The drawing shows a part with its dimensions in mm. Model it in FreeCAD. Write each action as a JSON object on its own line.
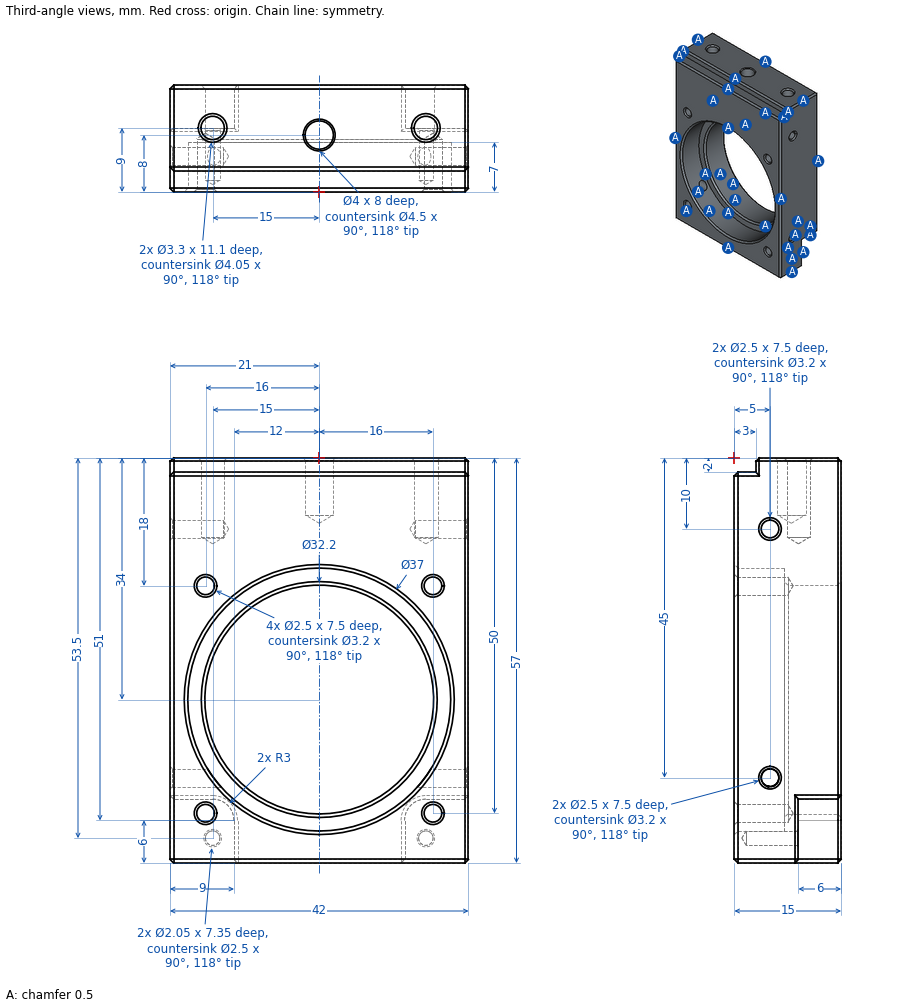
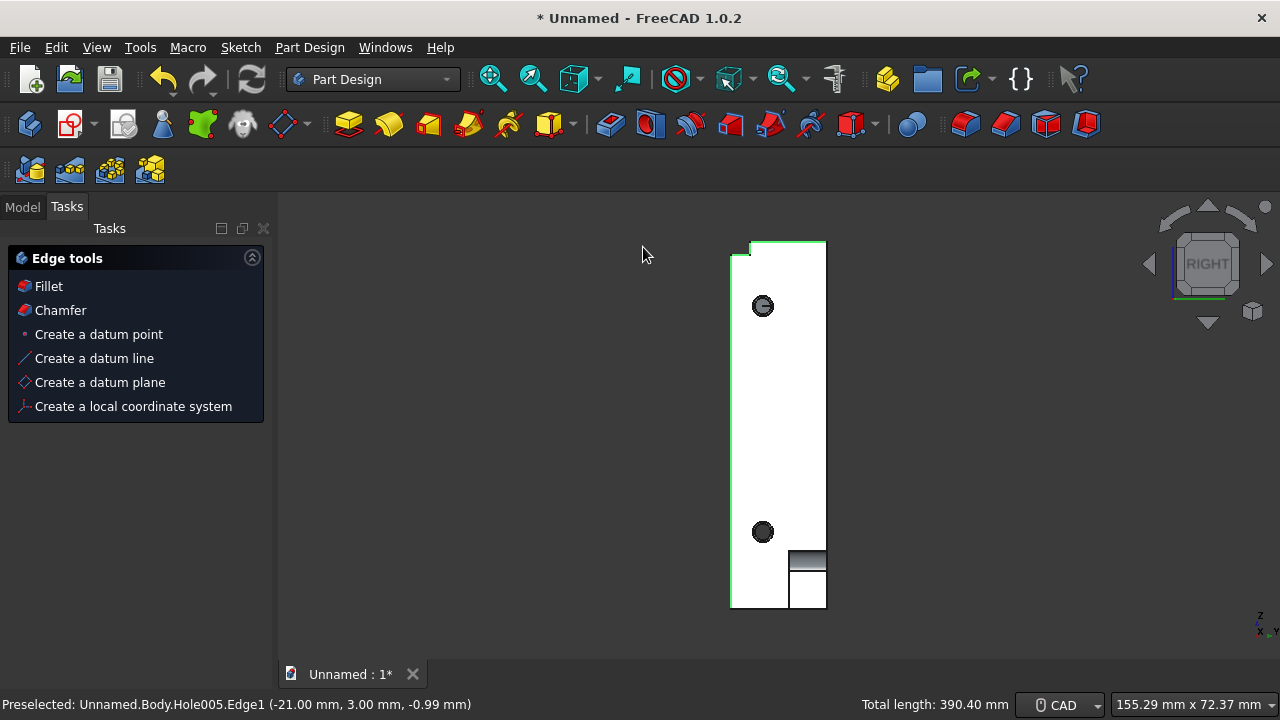
{"action": "left_click", "coordinate": [789, 579], "text": "ctrl"}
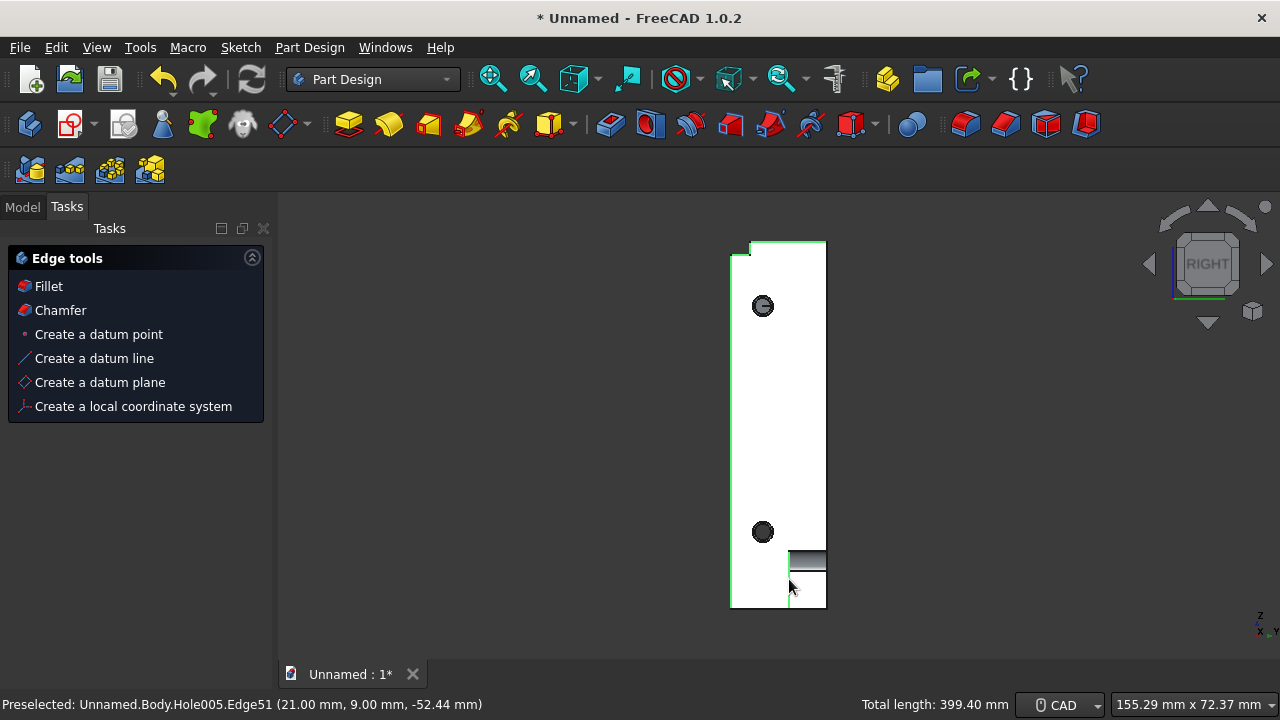
{"action": "left_click", "coordinate": [808, 550], "text": "ctrl"}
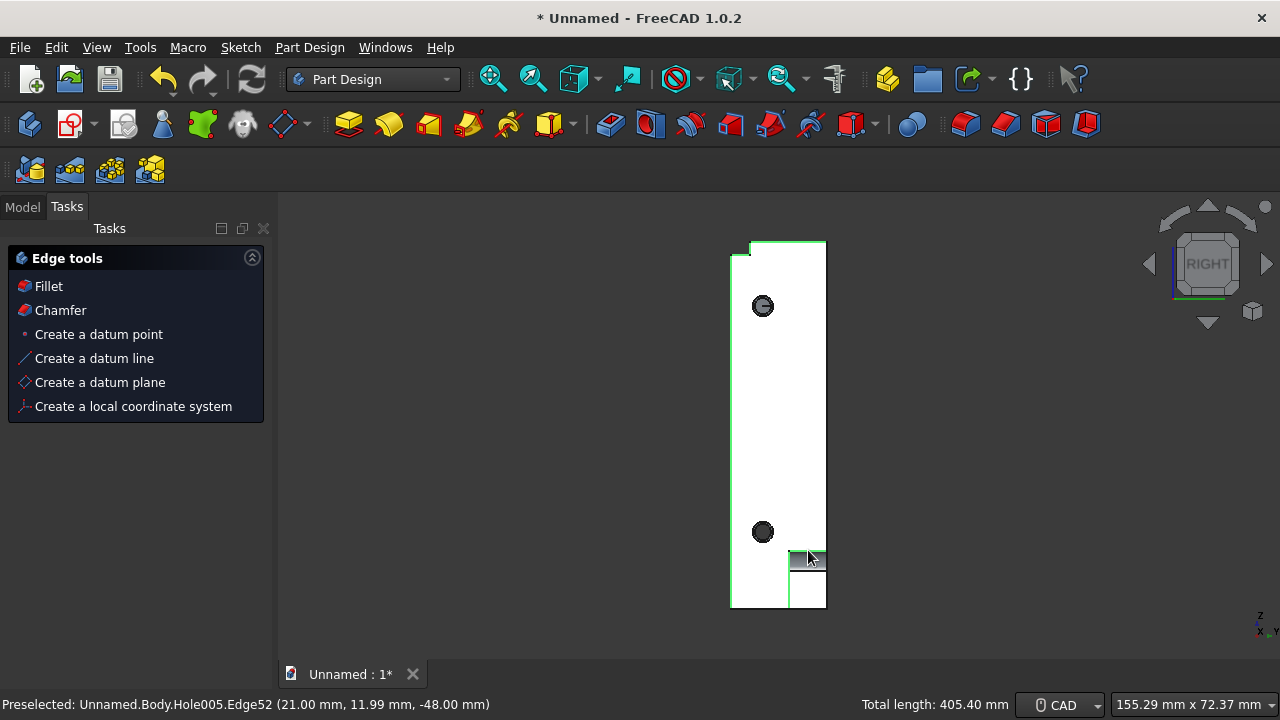
{"action": "key", "text": "5"}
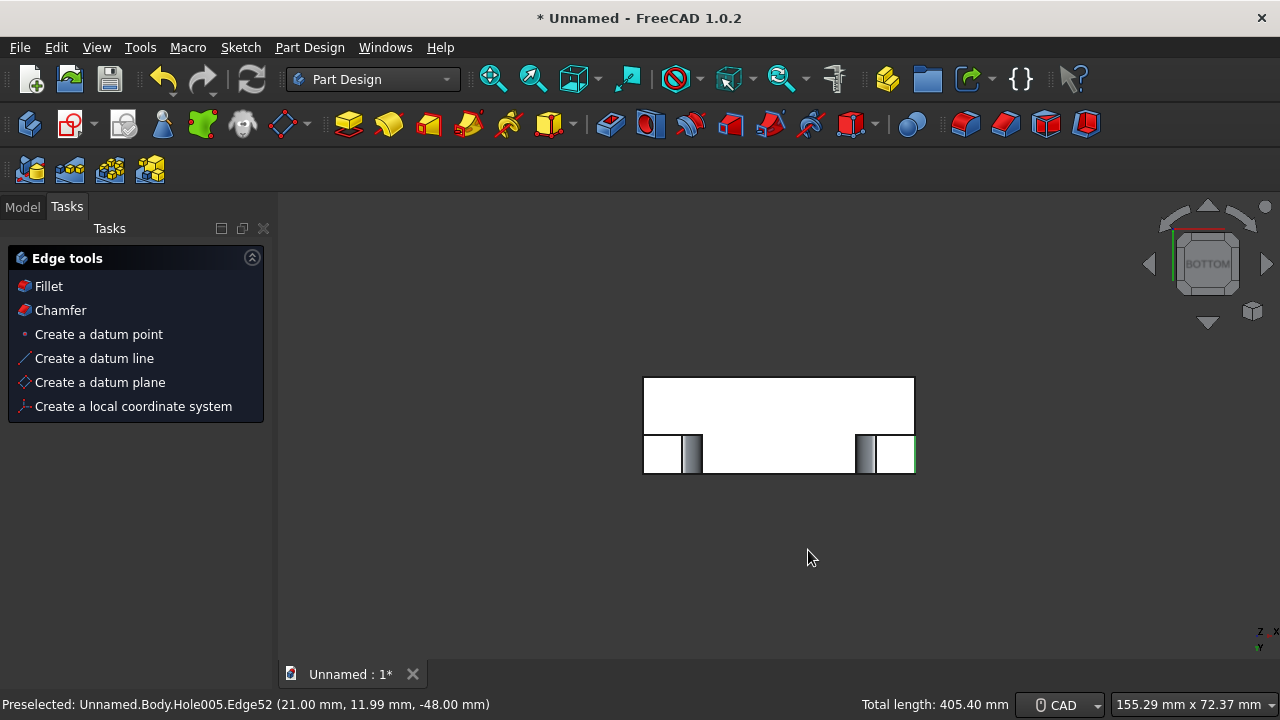
{"action": "key", "text": "v f"}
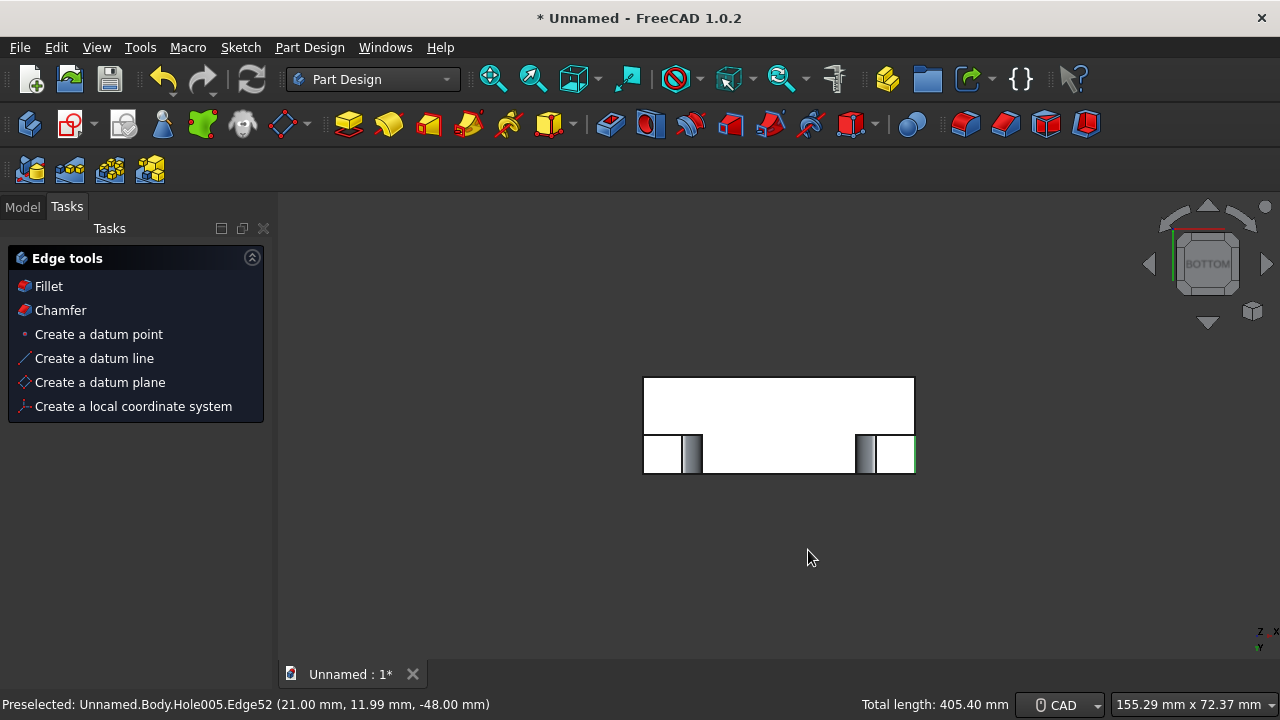
{"action": "left_click", "coordinate": [779, 424], "text": "ctrl"}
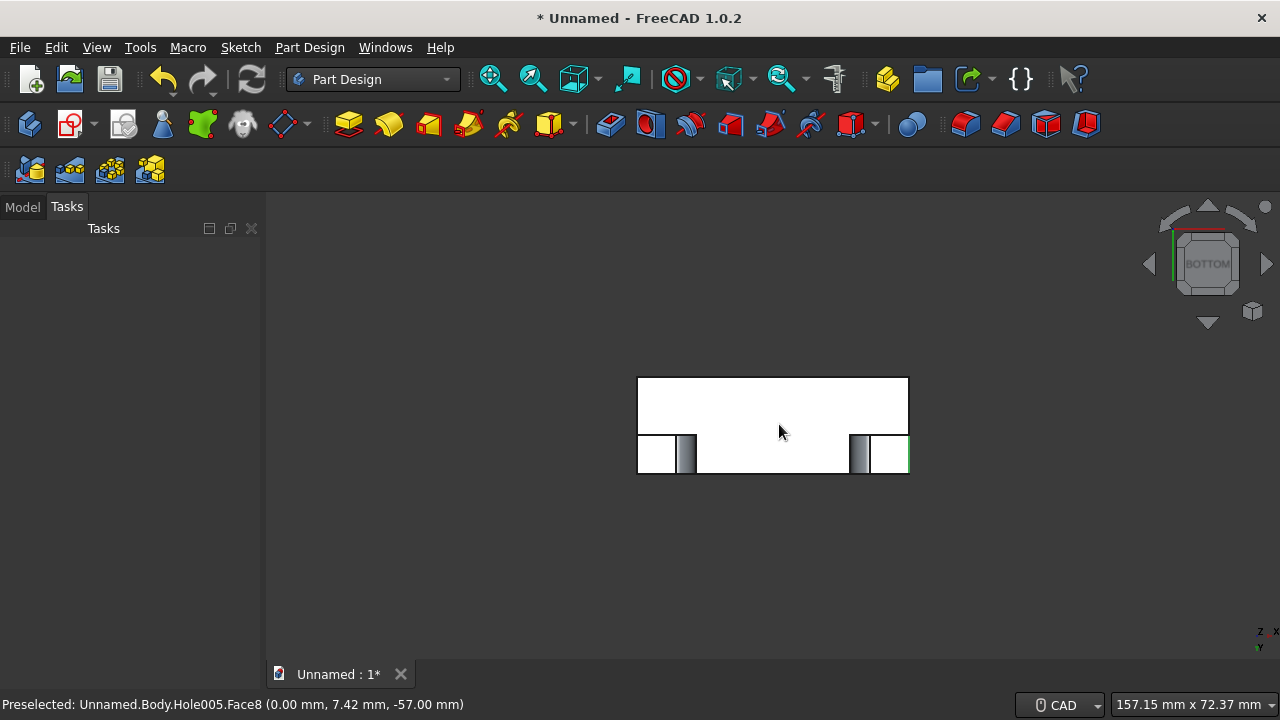
{"action": "left_click", "coordinate": [637, 454], "text": "ctrl"}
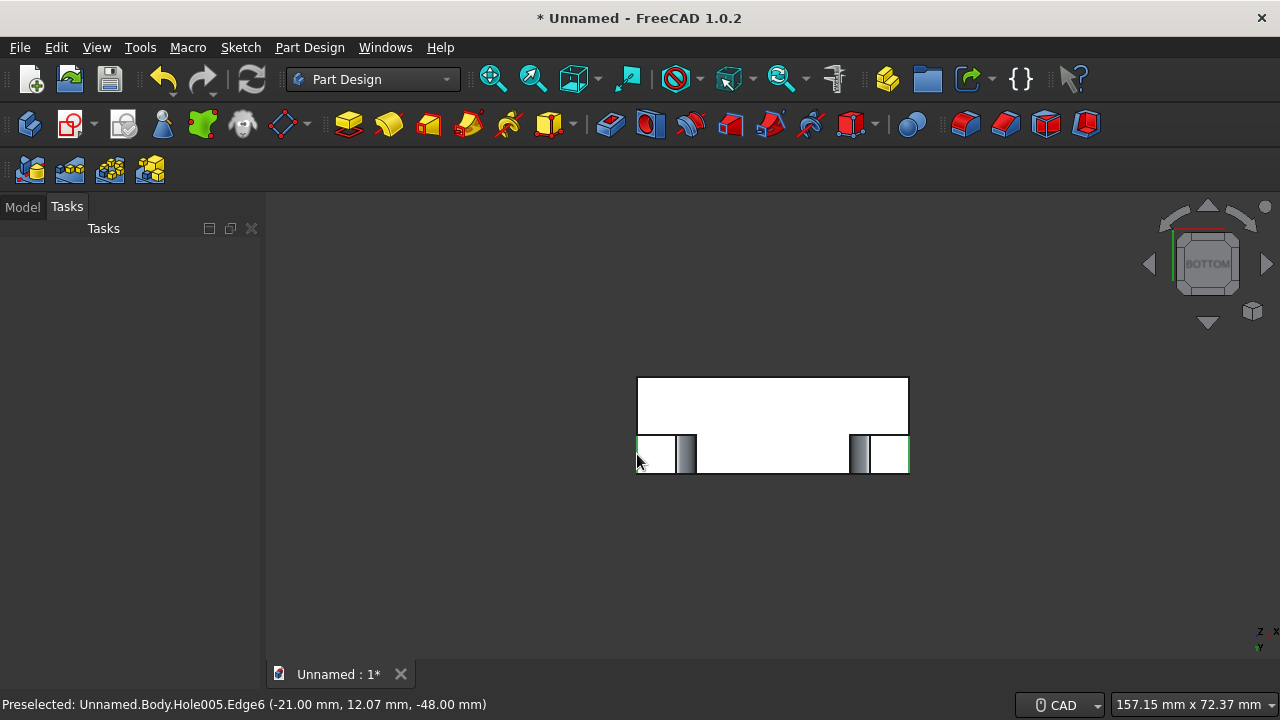
{"action": "key", "text": "4"}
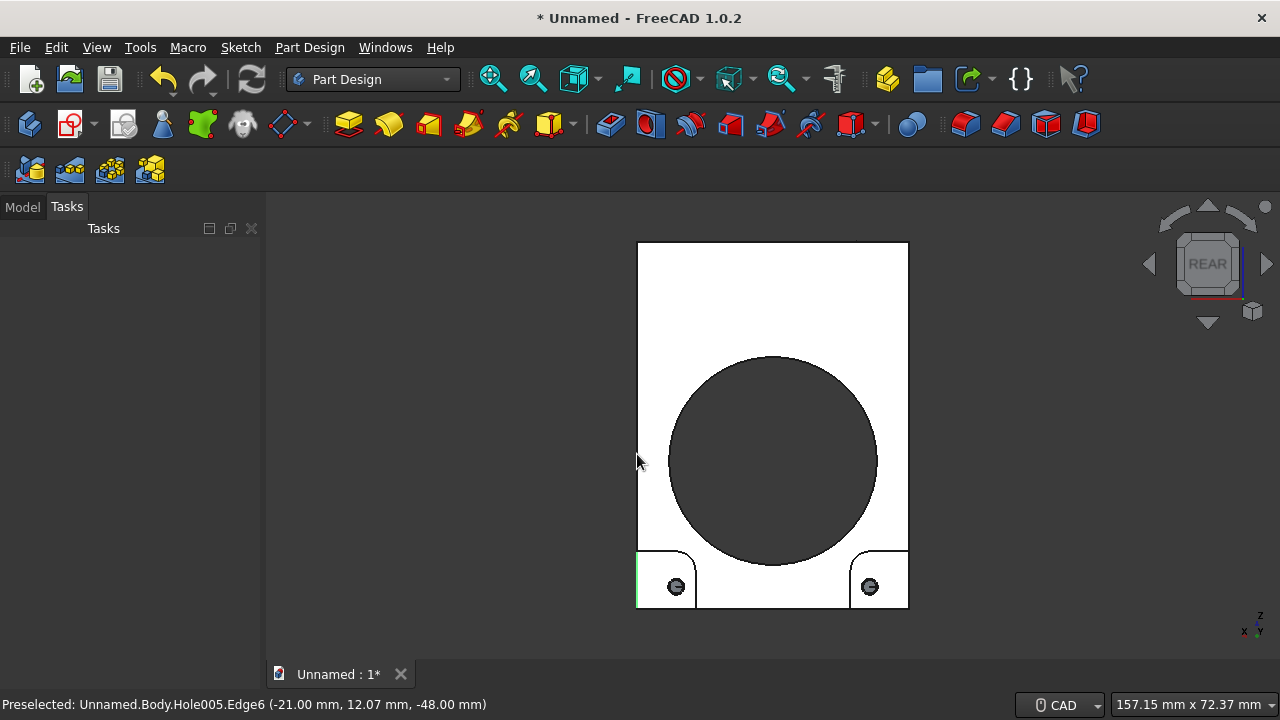
{"action": "left_click", "coordinate": [696, 319], "text": "ctrl"}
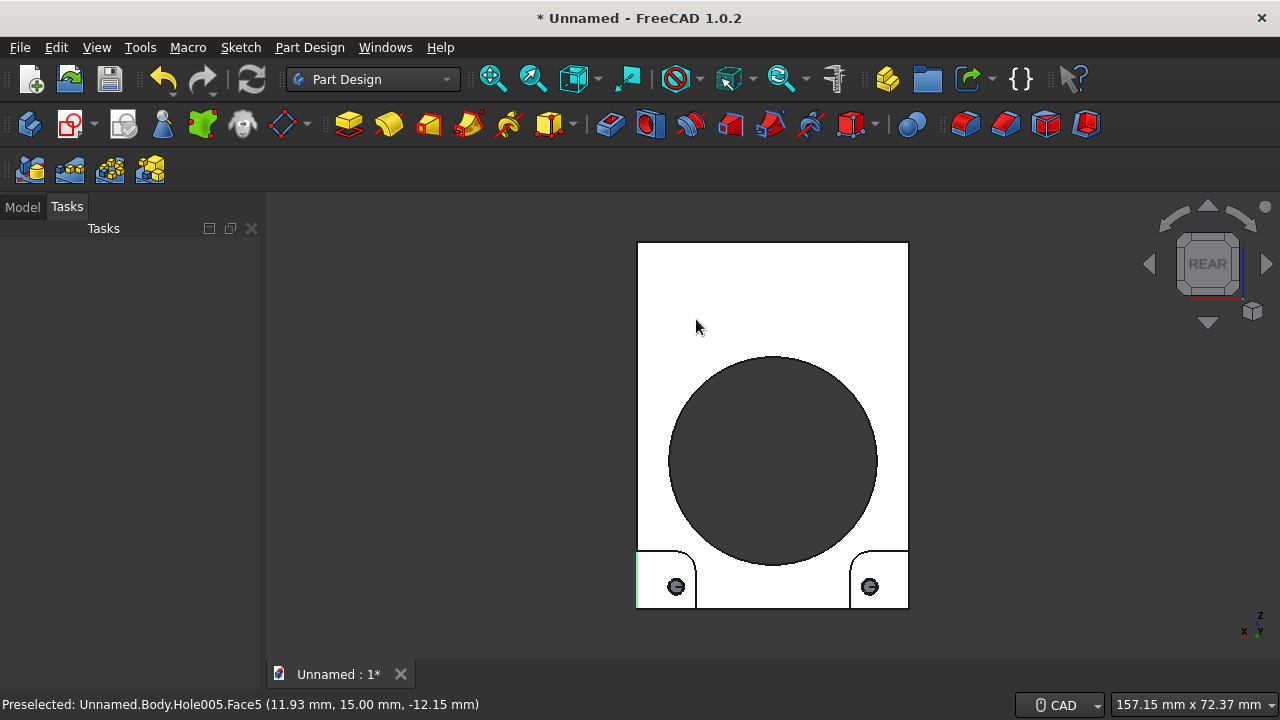
{"action": "left_click", "coordinate": [909, 579], "text": "ctrl"}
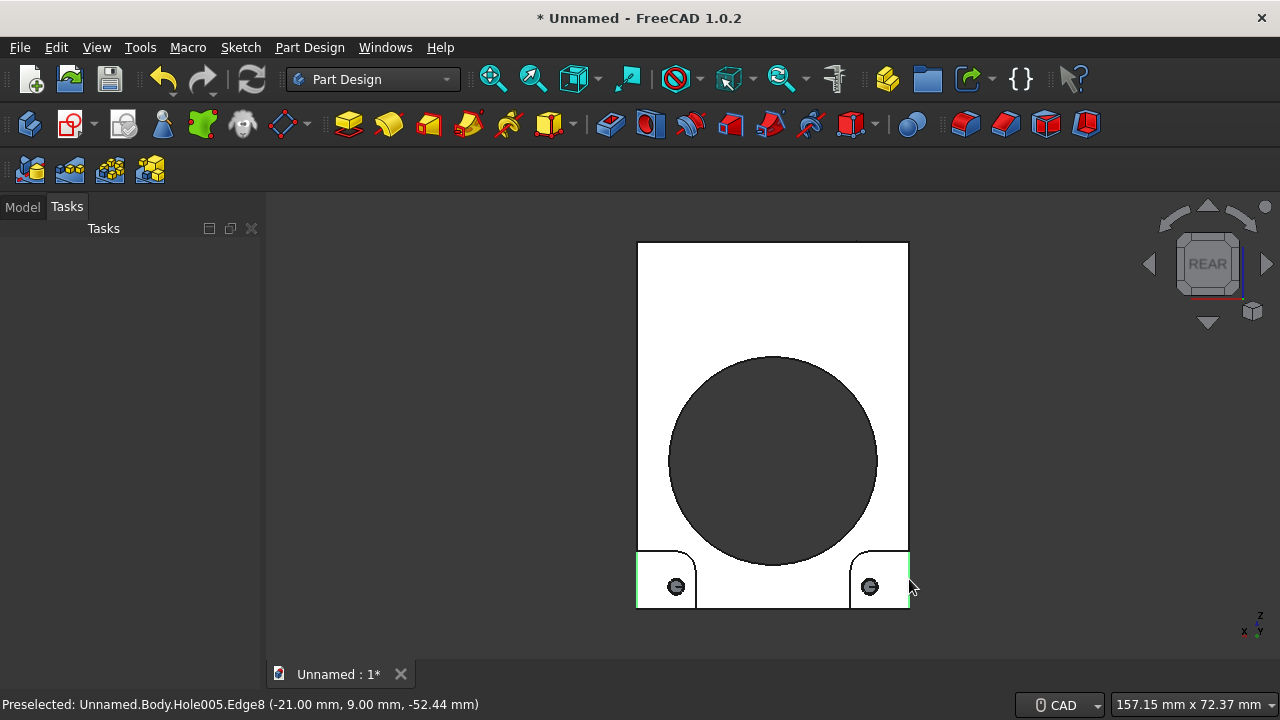
{"action": "key", "text": "6"}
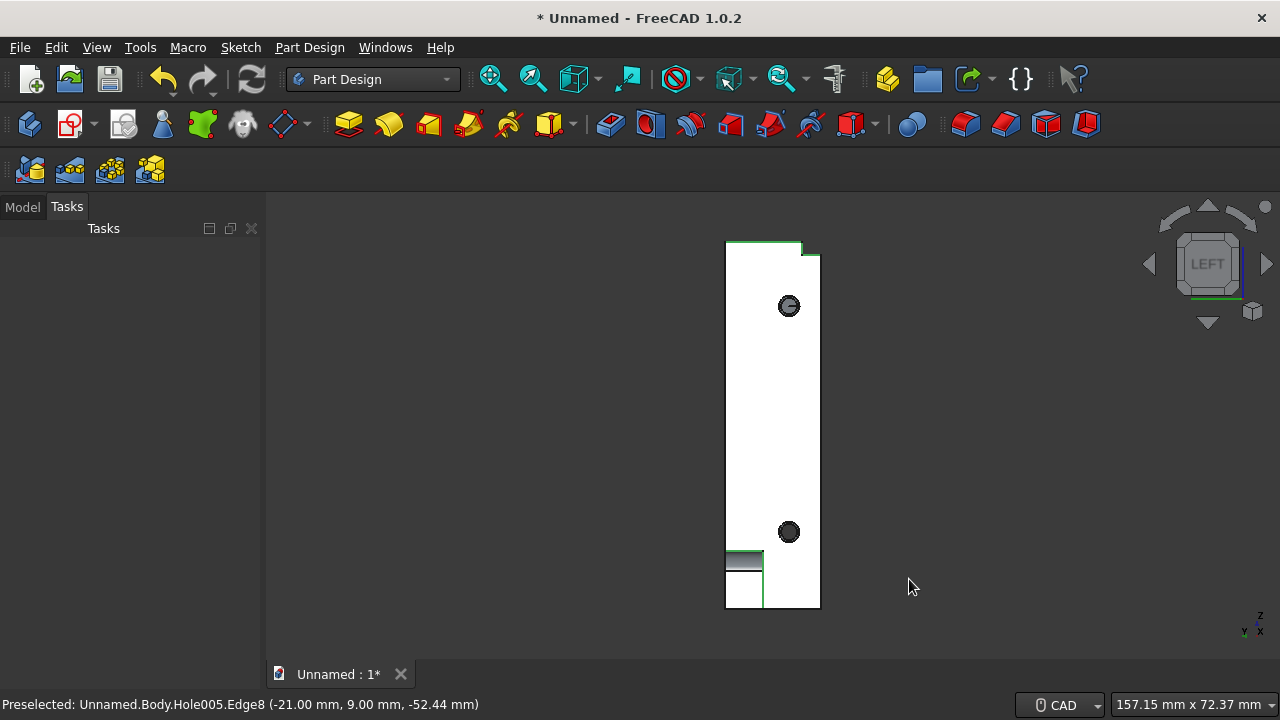
{"action": "left_click", "coordinate": [821, 431], "text": "ctrl"}